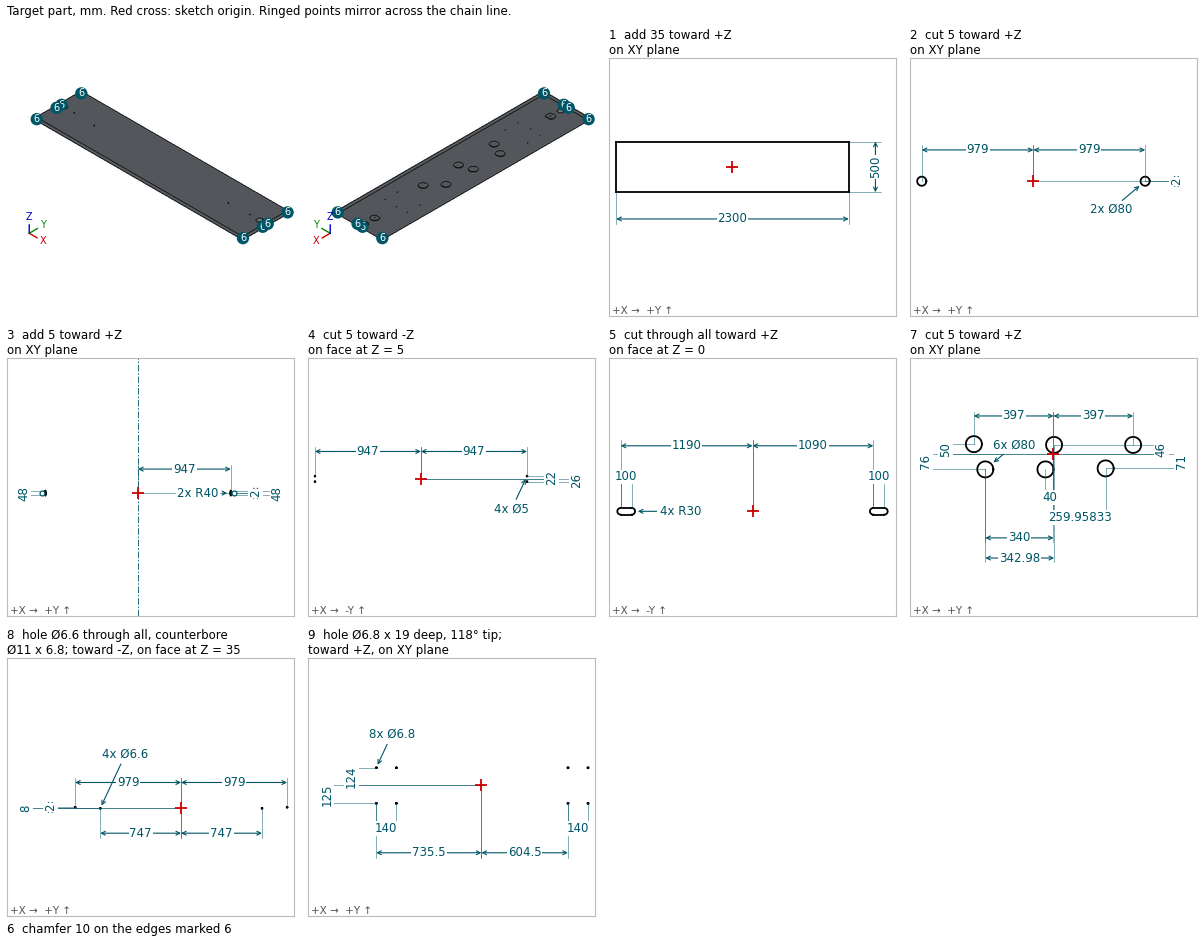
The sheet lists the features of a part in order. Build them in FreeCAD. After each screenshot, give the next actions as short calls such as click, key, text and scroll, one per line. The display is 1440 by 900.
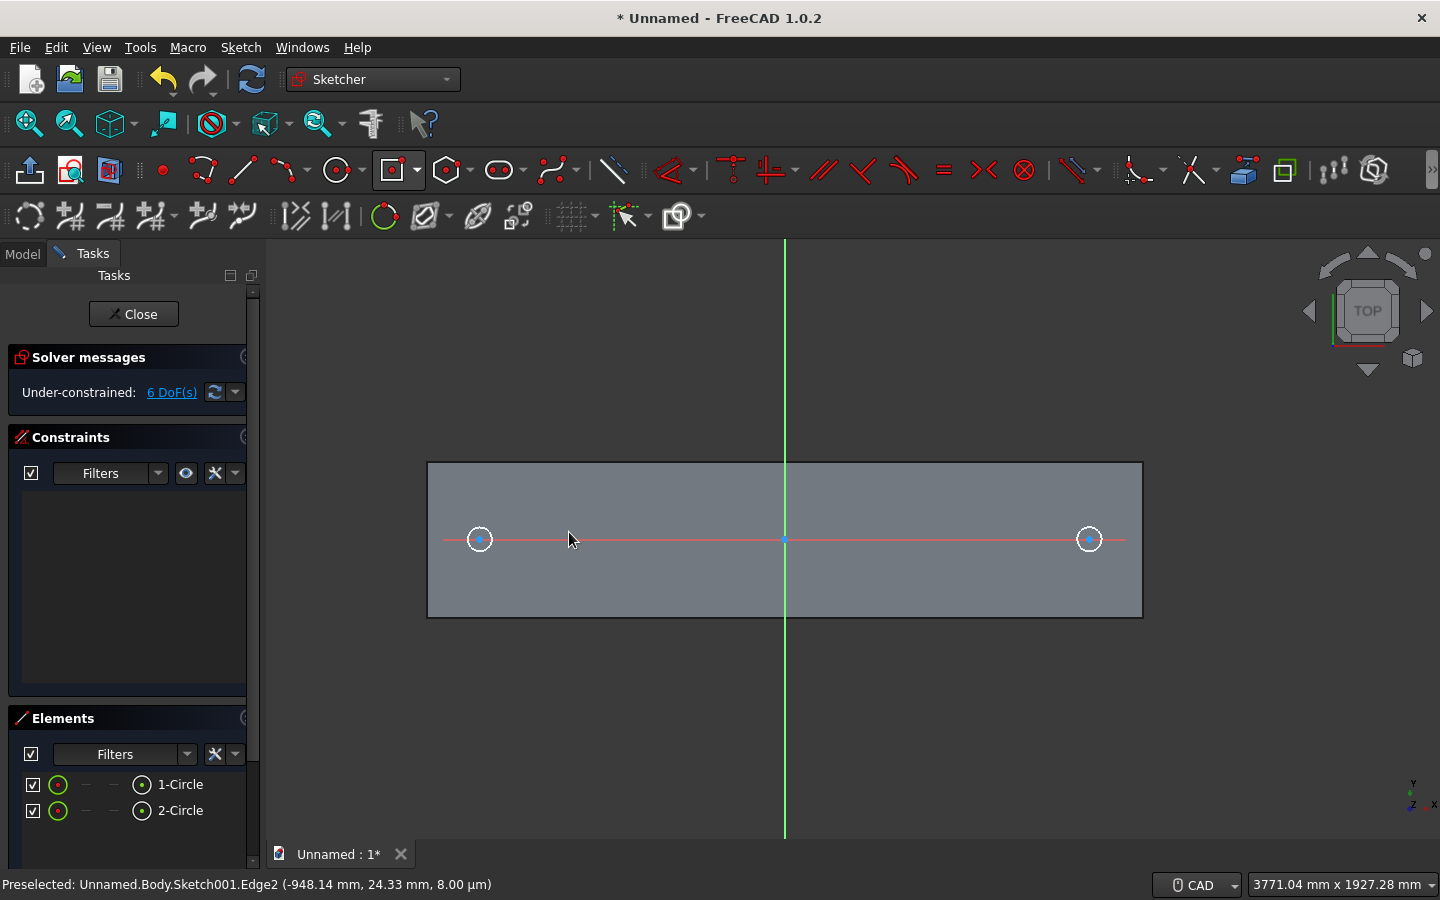
scroll(1098, 531, up, 3)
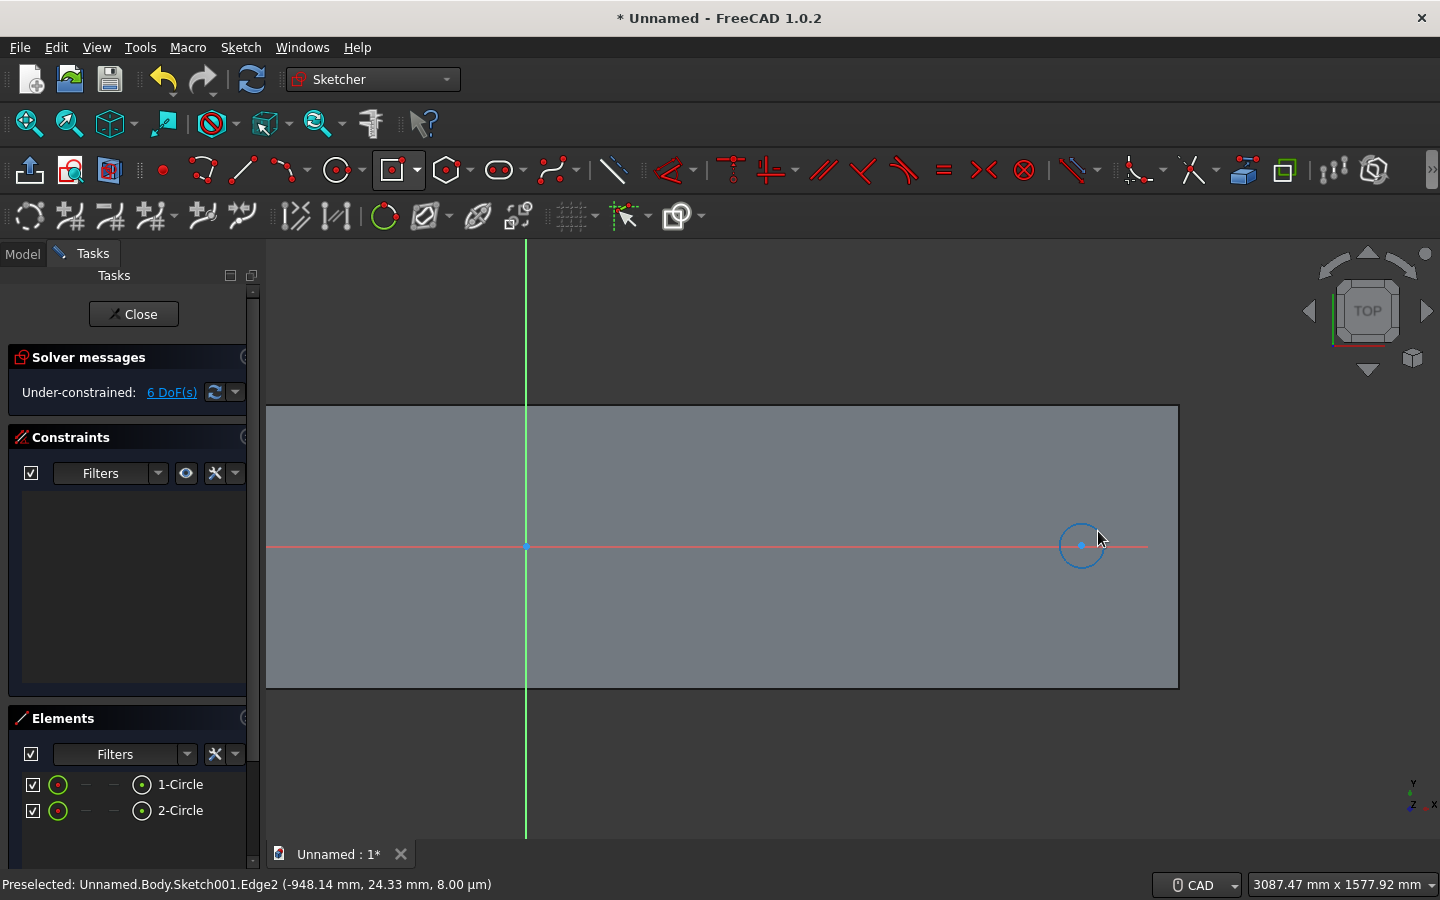
click(1097, 530)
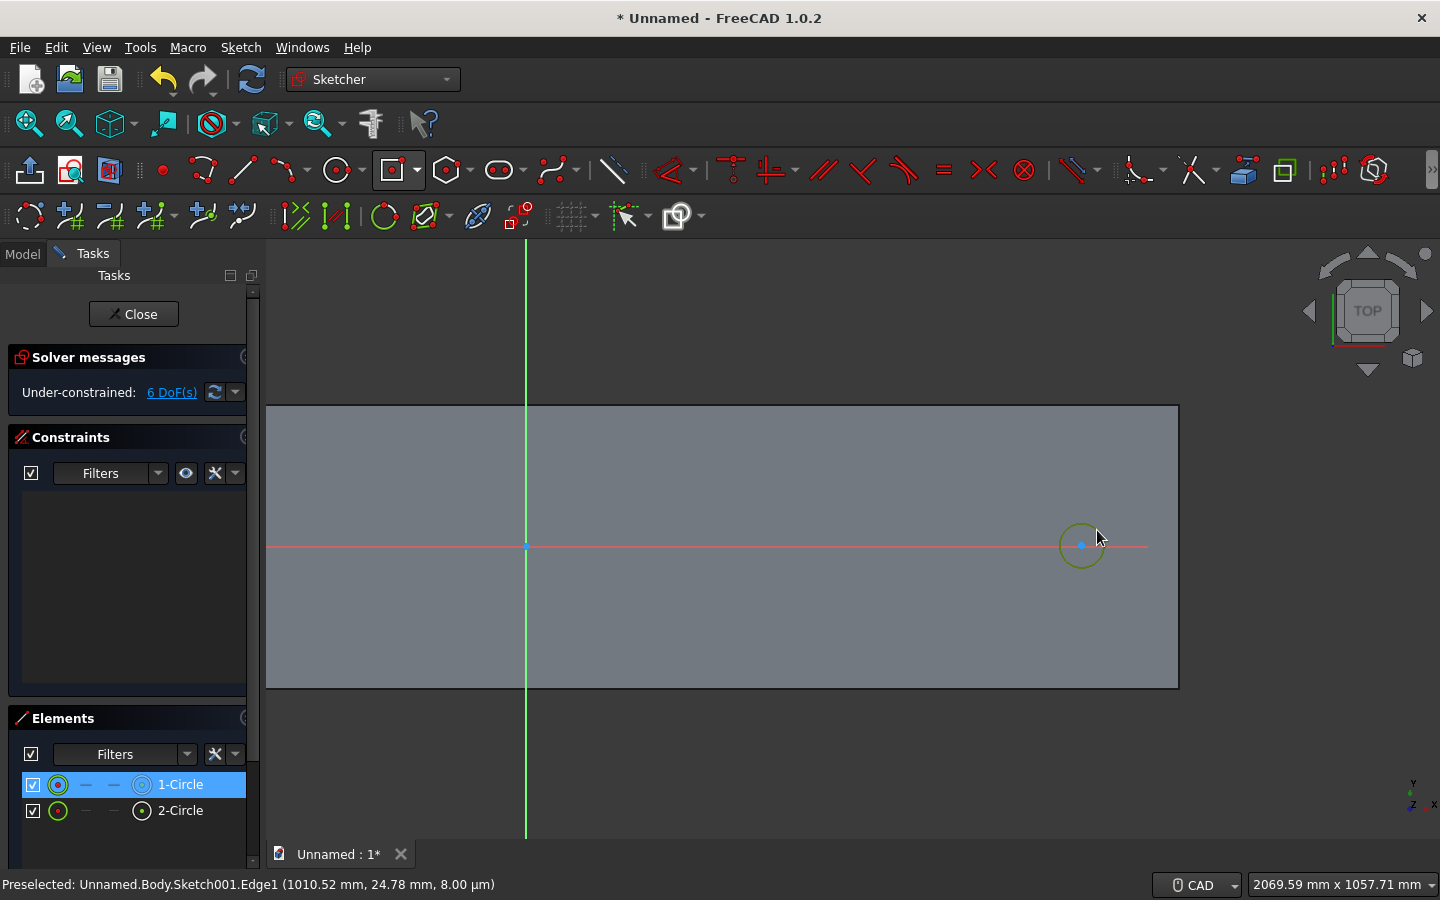
scroll(1098, 531, down, 3)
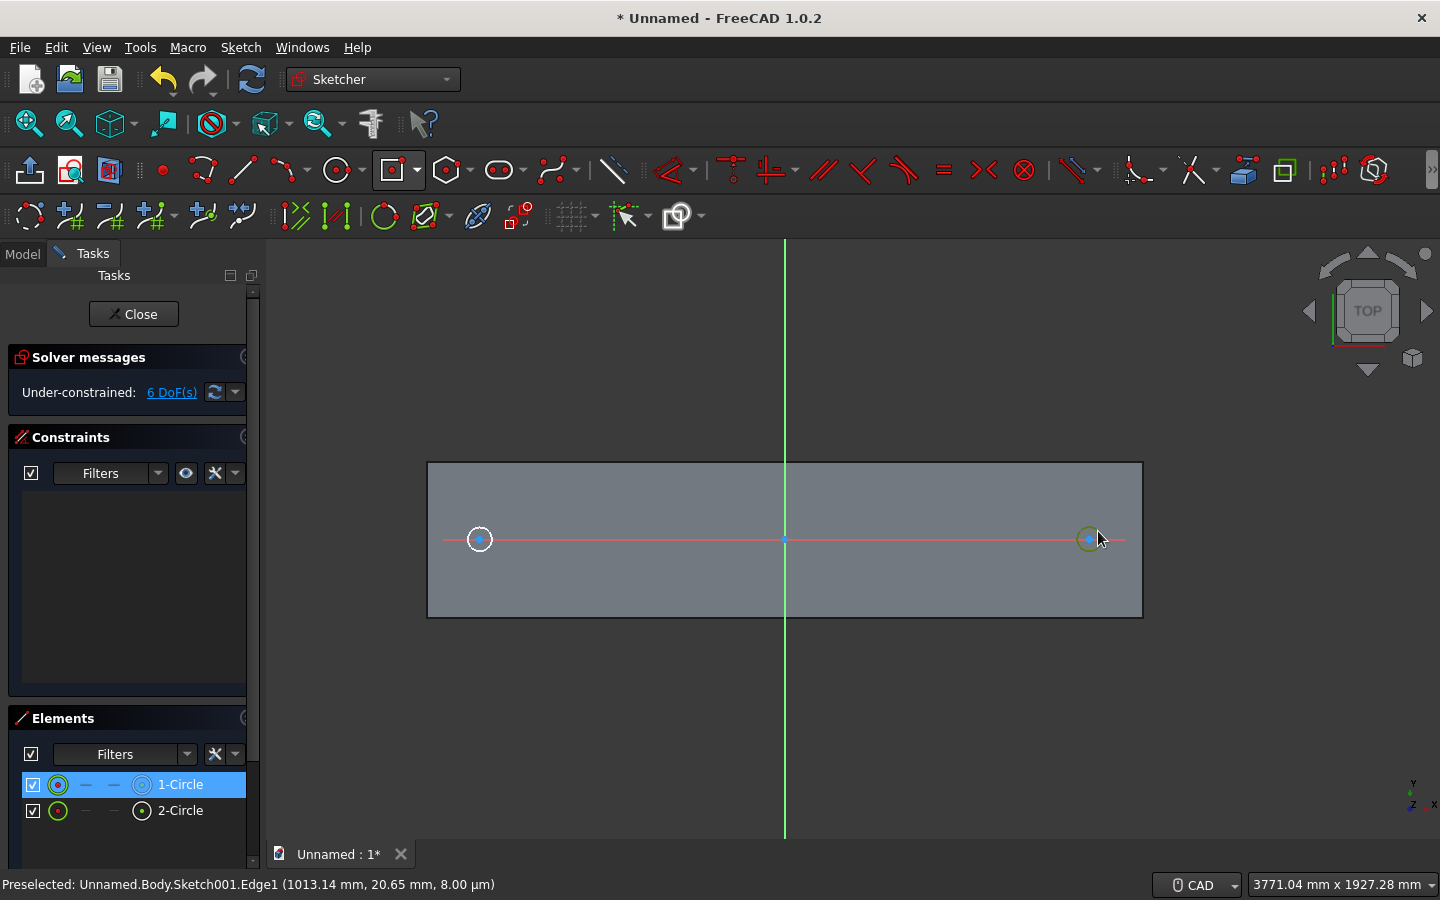
scroll(488, 531, up, 3)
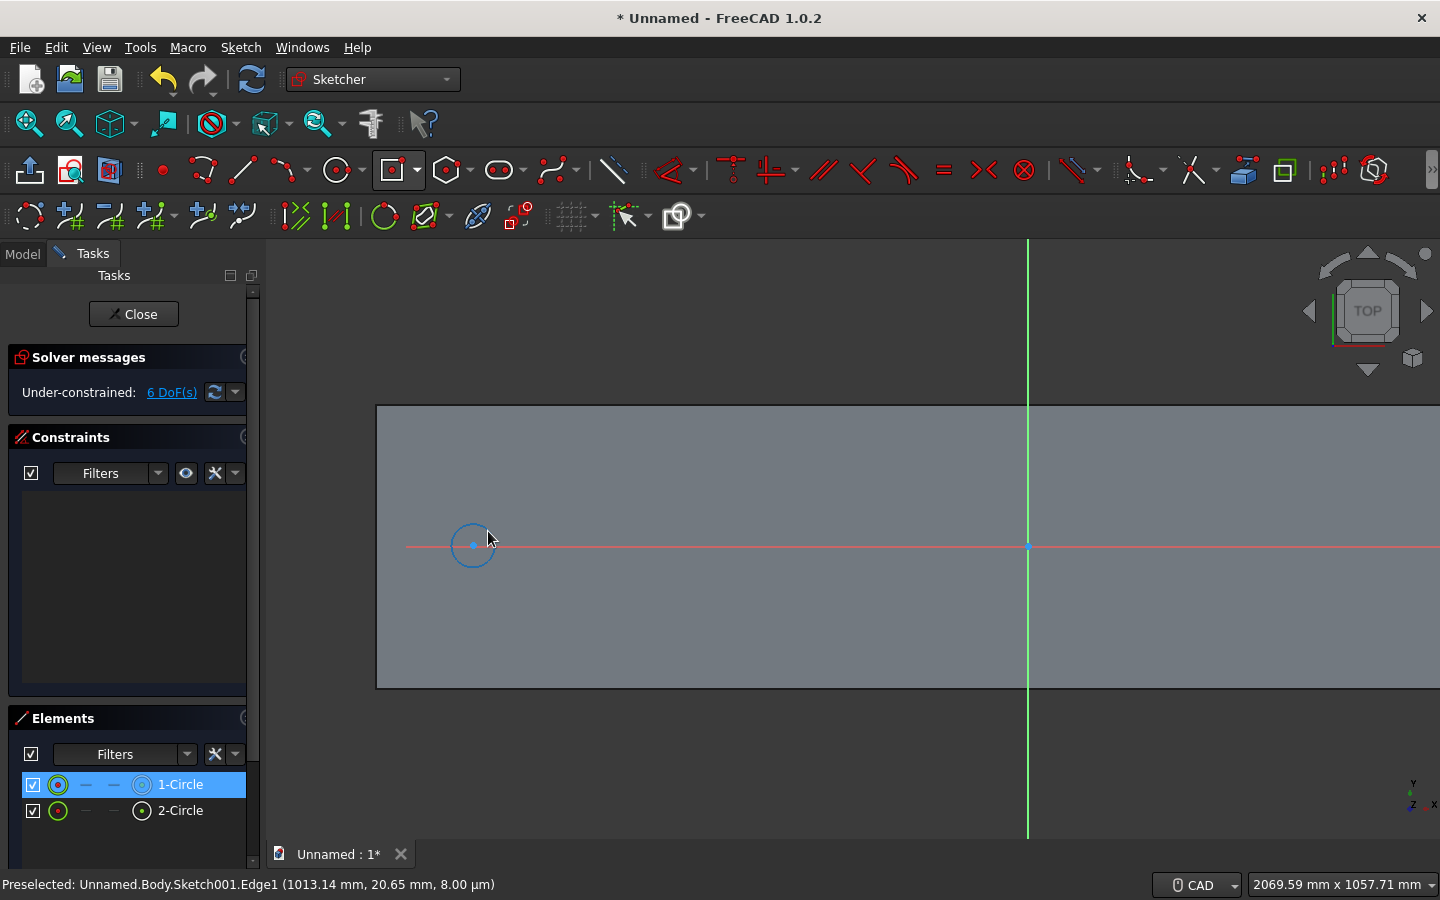
click(488, 530)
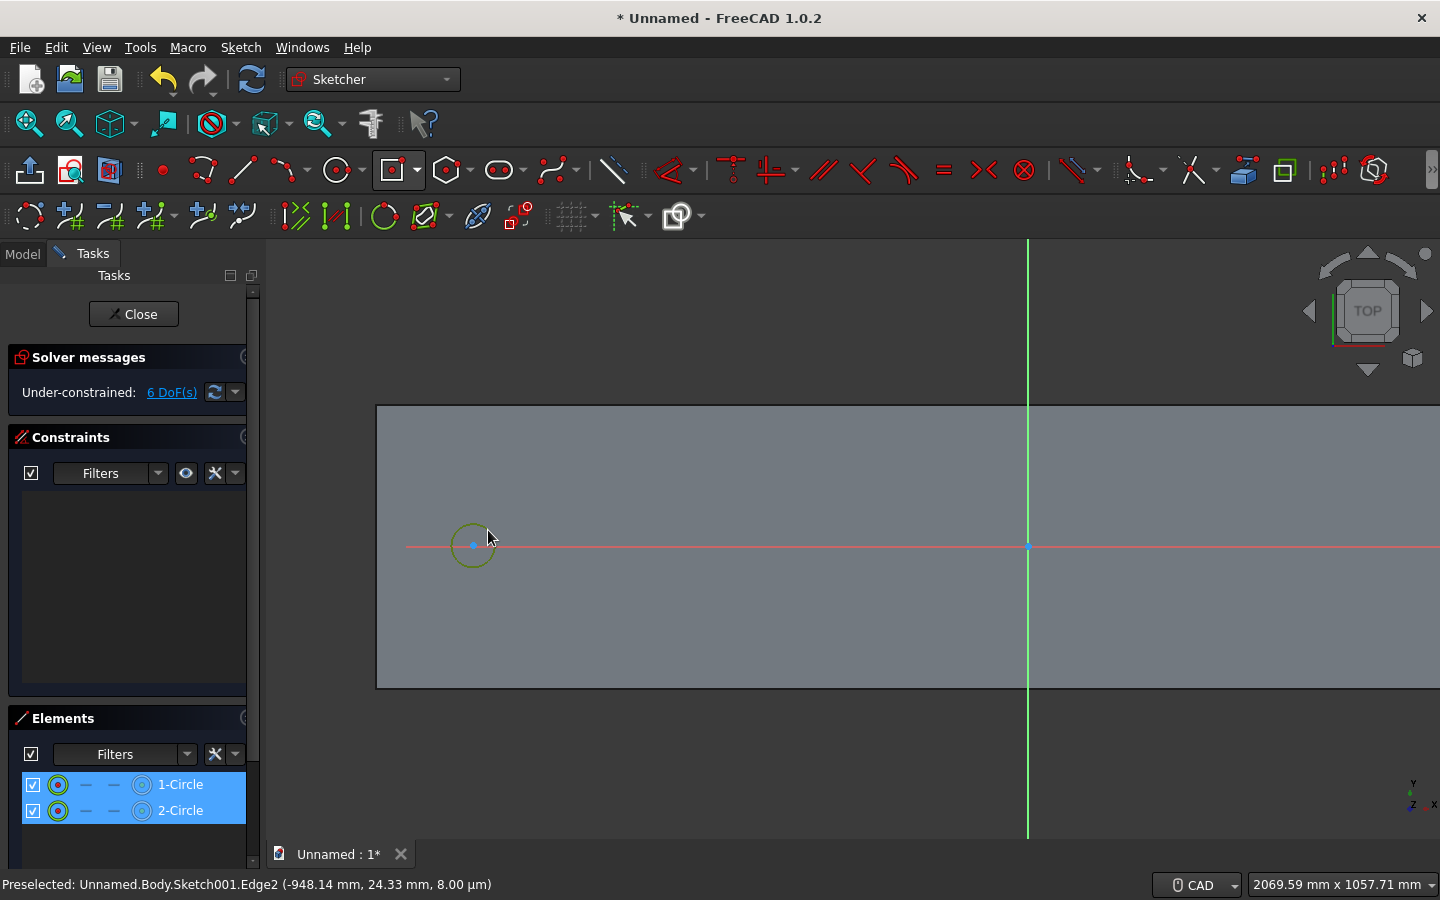
click(944, 170)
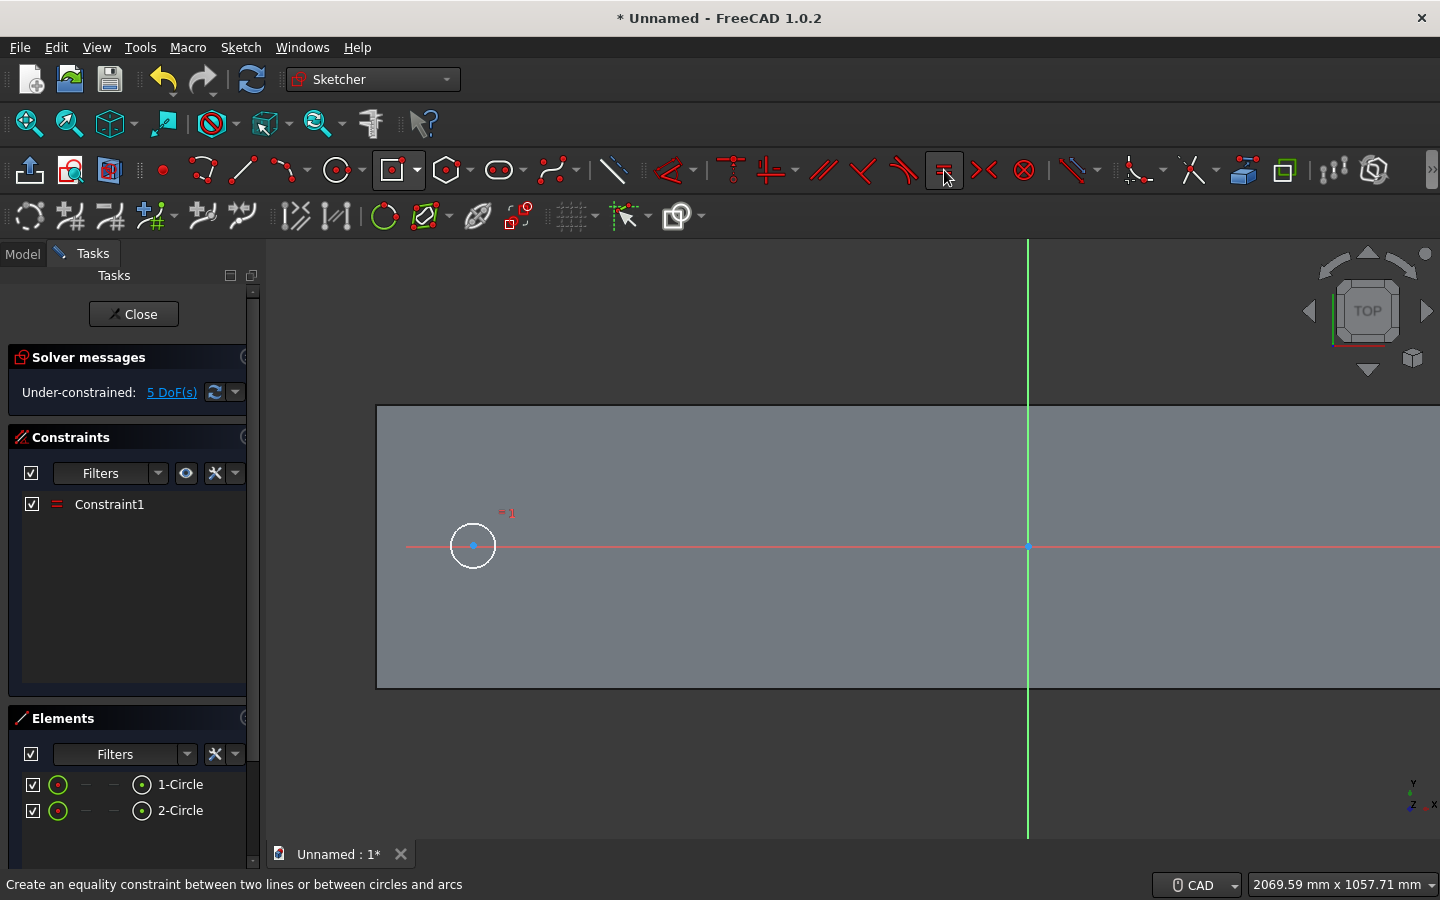
scroll(488, 531, down, 3)